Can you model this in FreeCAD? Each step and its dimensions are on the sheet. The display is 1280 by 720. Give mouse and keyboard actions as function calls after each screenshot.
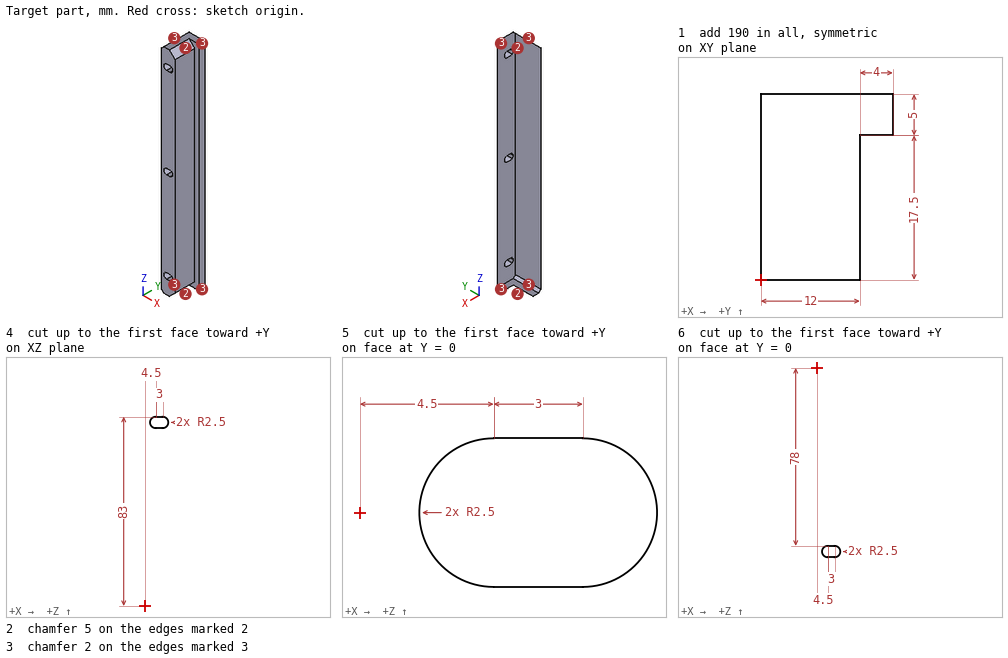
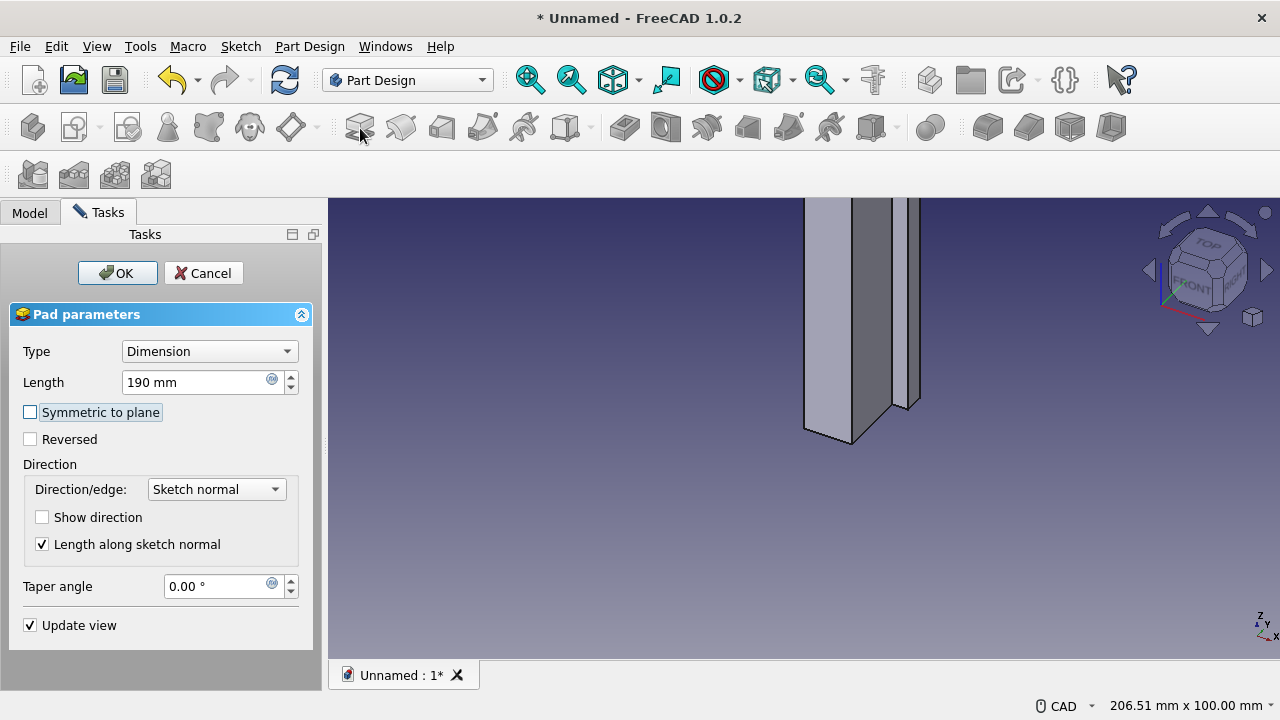
click(31, 412)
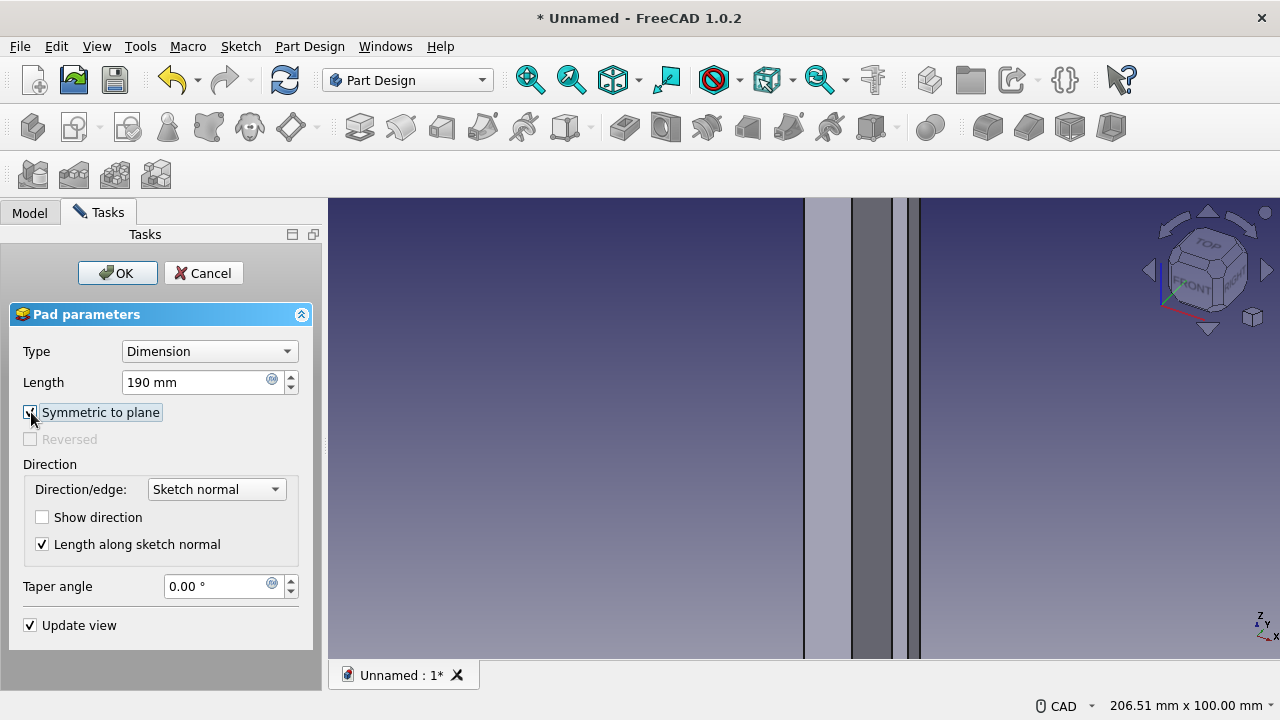
click(118, 273)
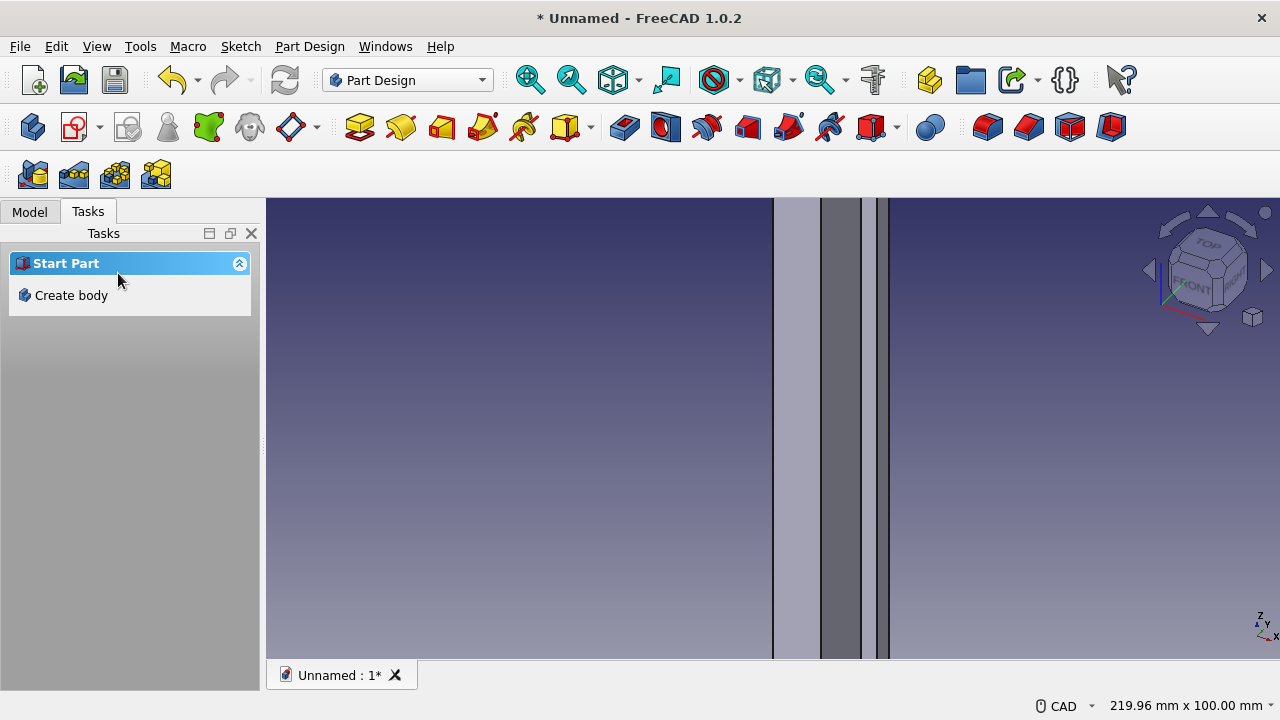
click(531, 80)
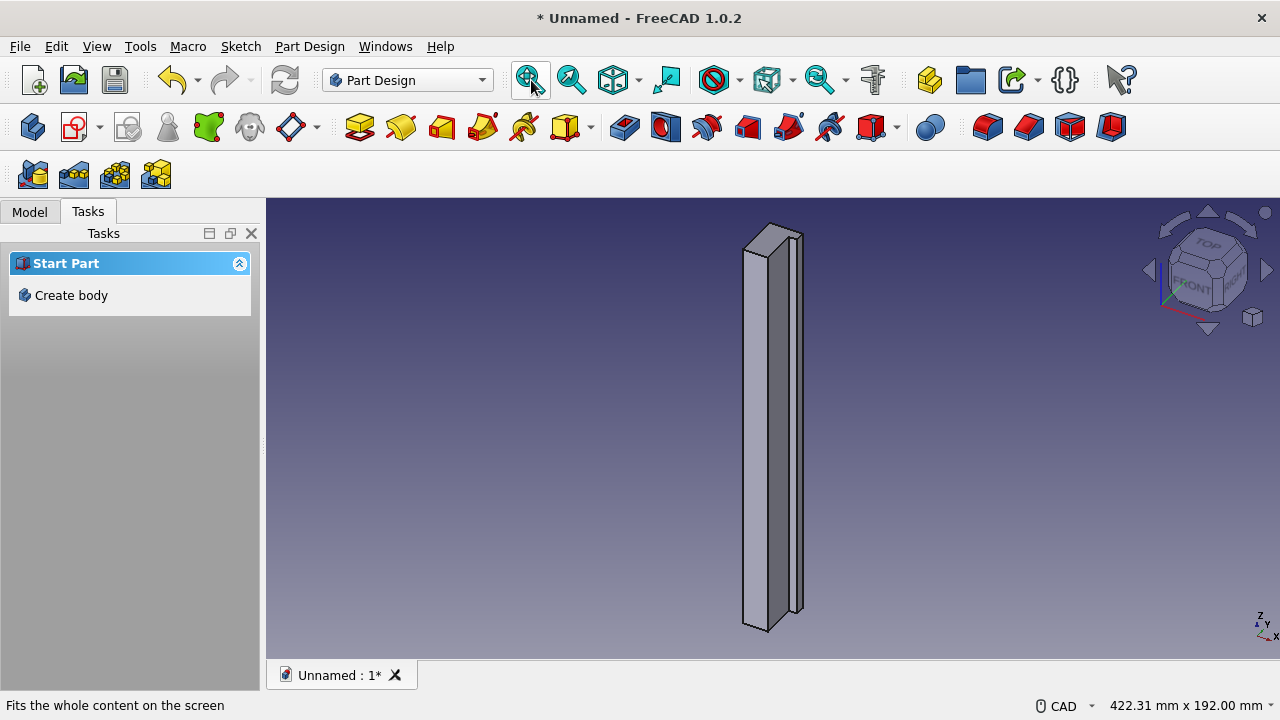
click(778, 246)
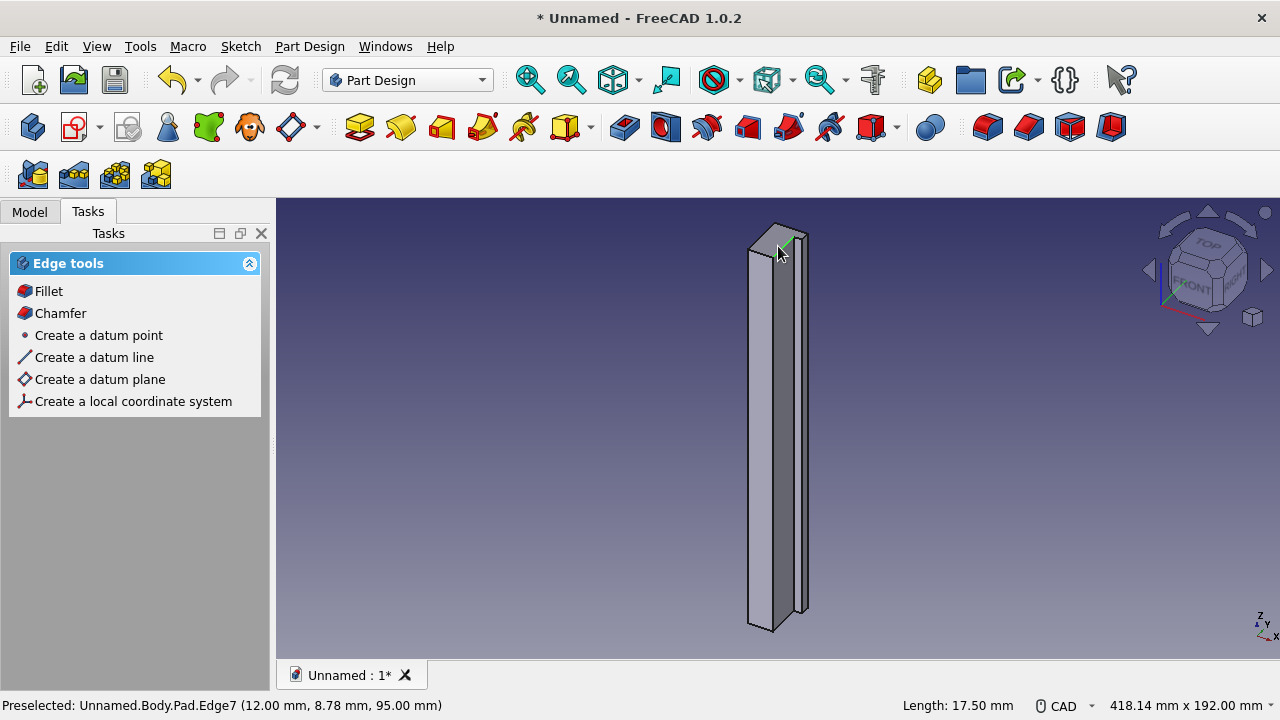
key(0)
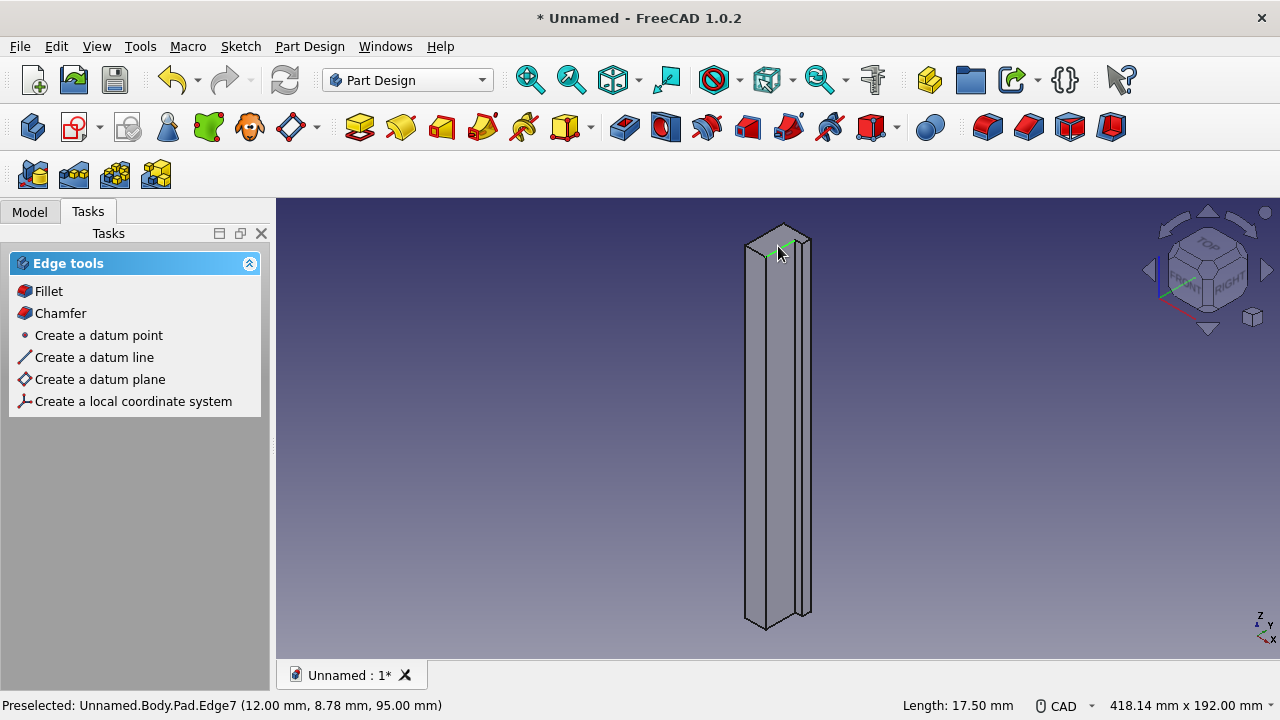
key(2)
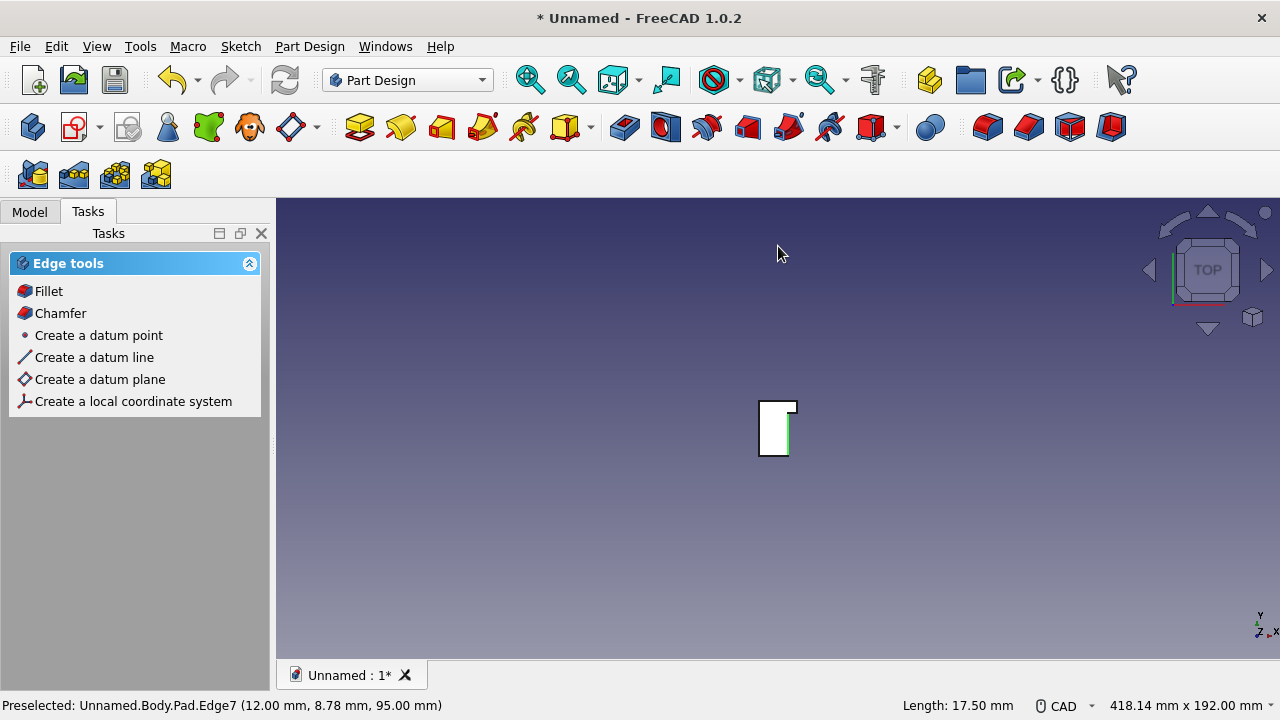
click(531, 80)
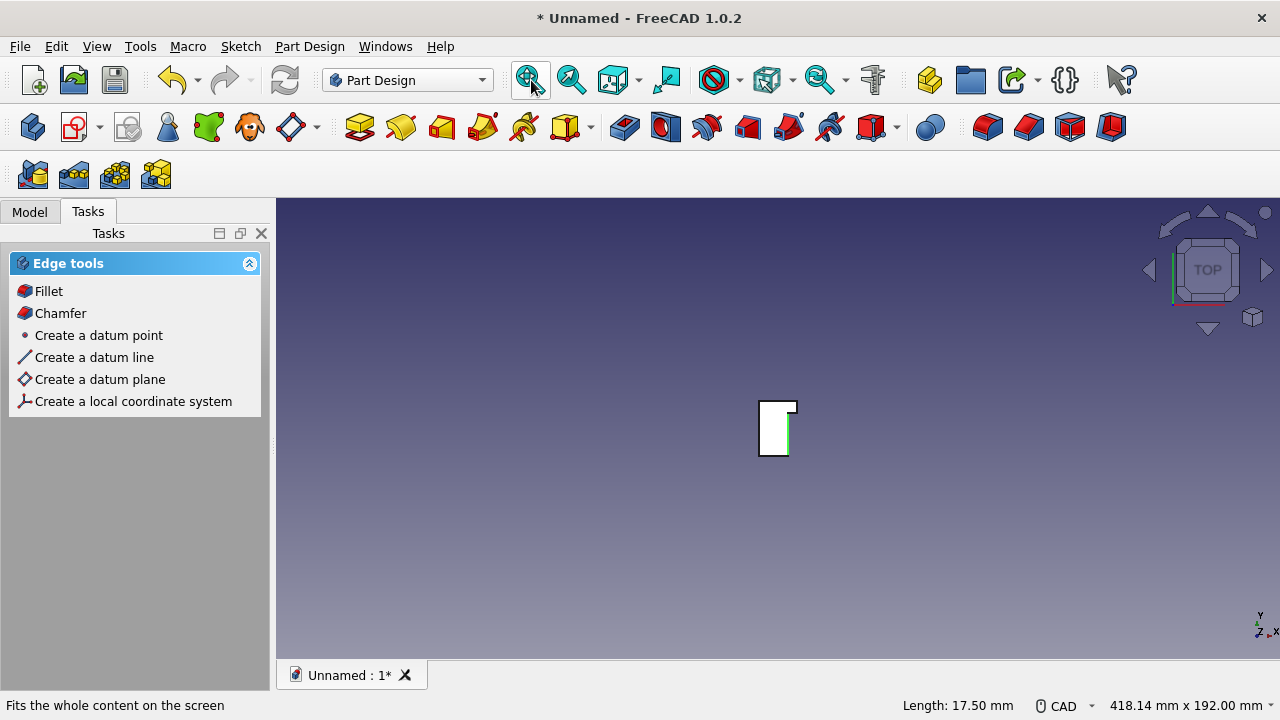
key(1)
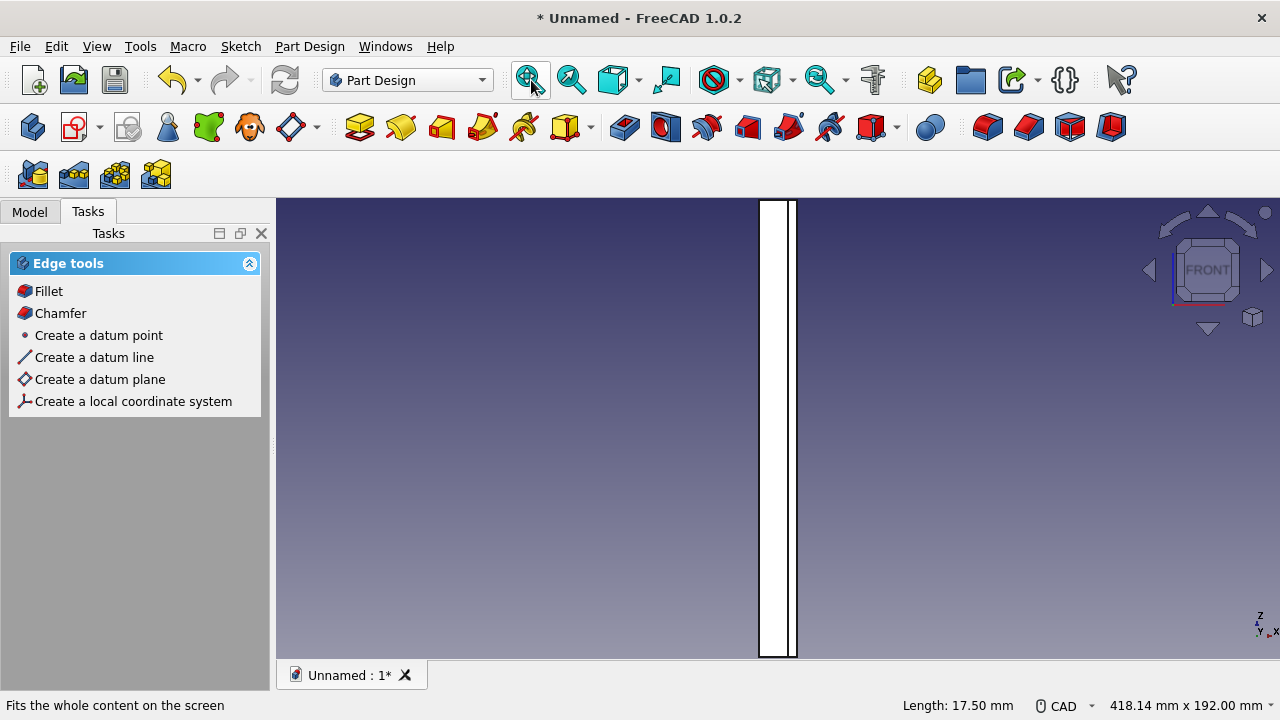
key(3)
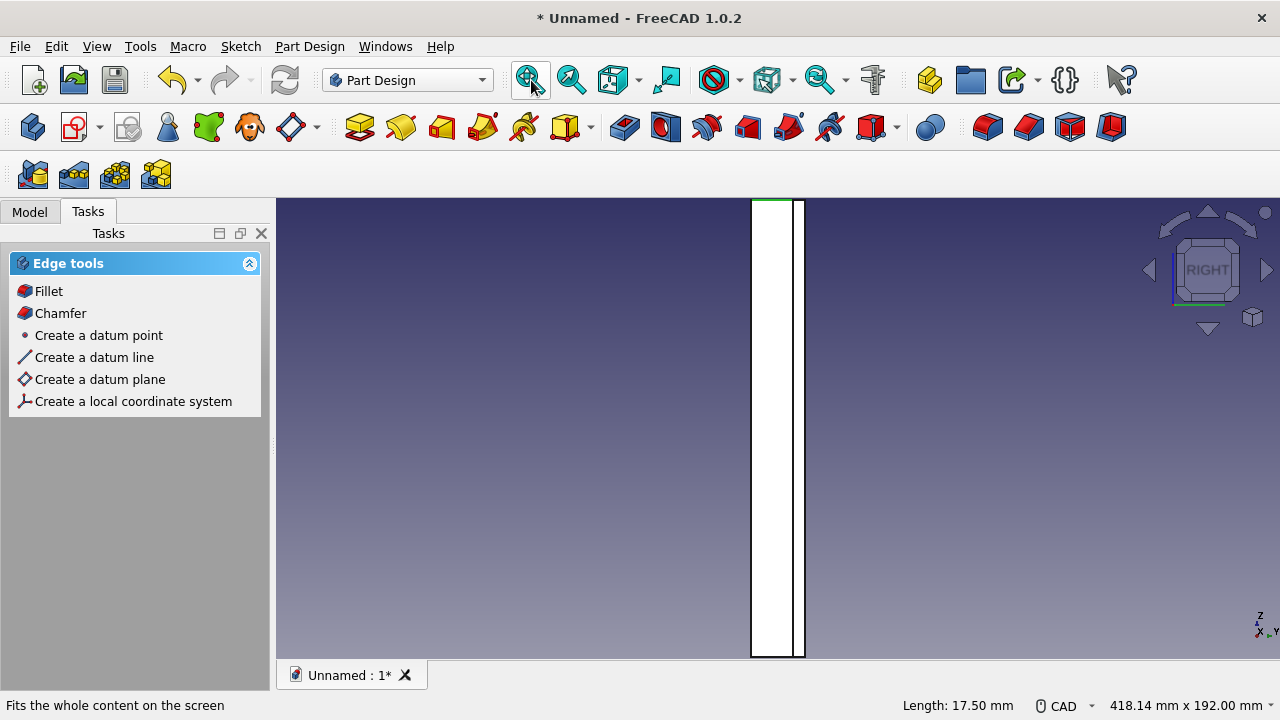
key(5)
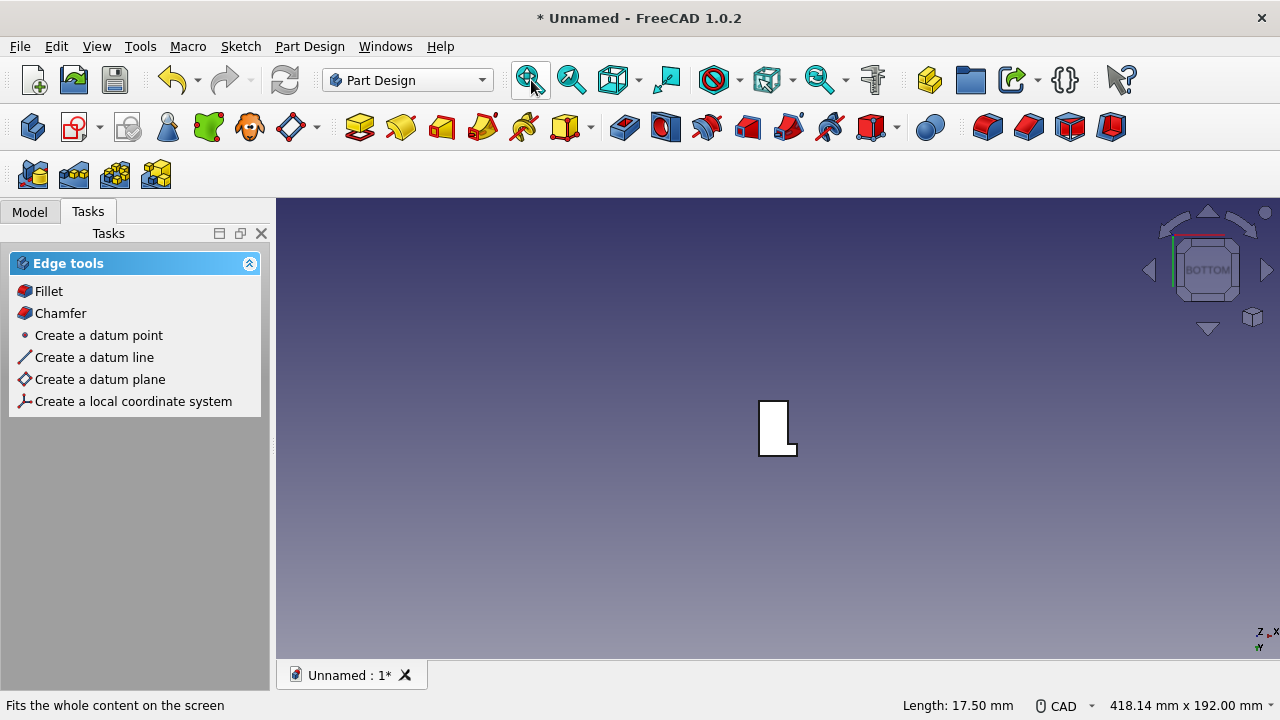
click(531, 80)